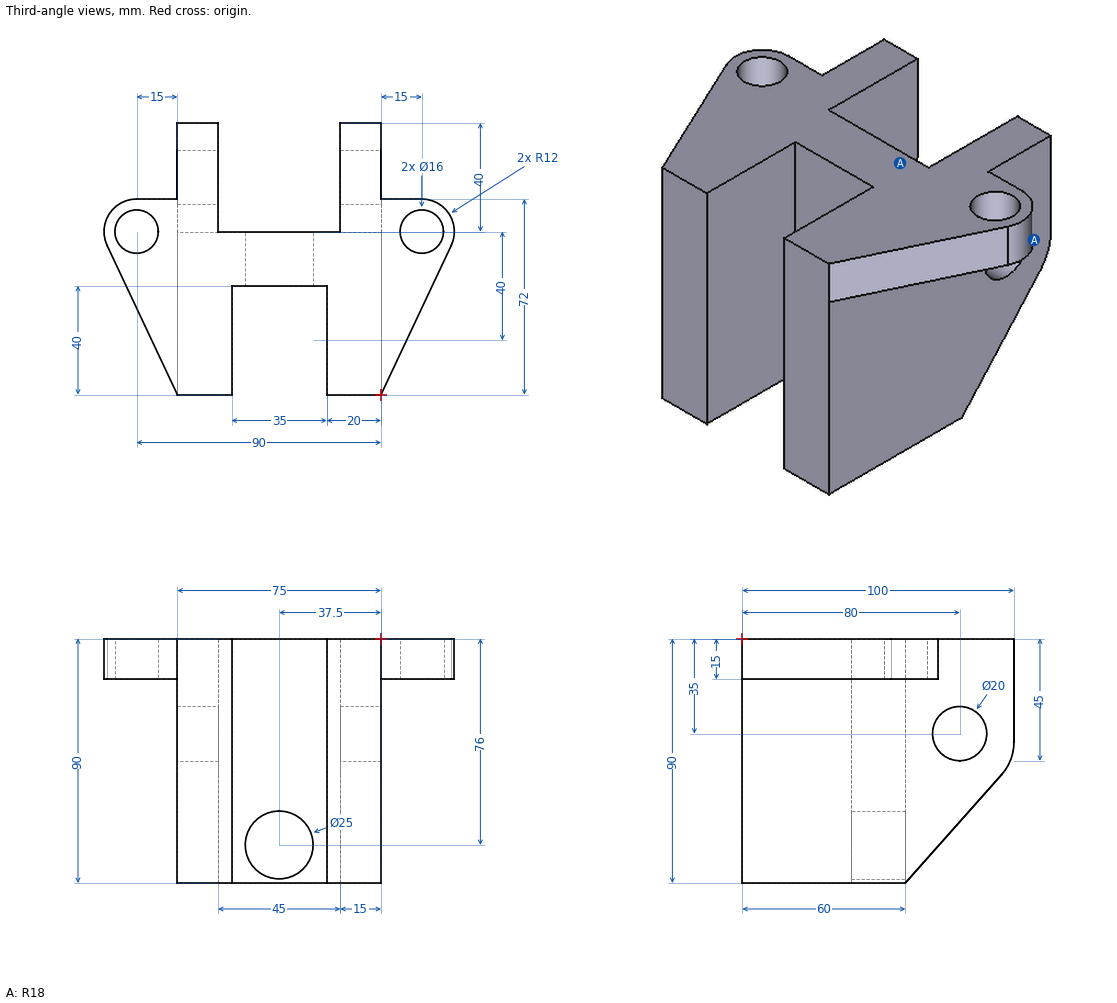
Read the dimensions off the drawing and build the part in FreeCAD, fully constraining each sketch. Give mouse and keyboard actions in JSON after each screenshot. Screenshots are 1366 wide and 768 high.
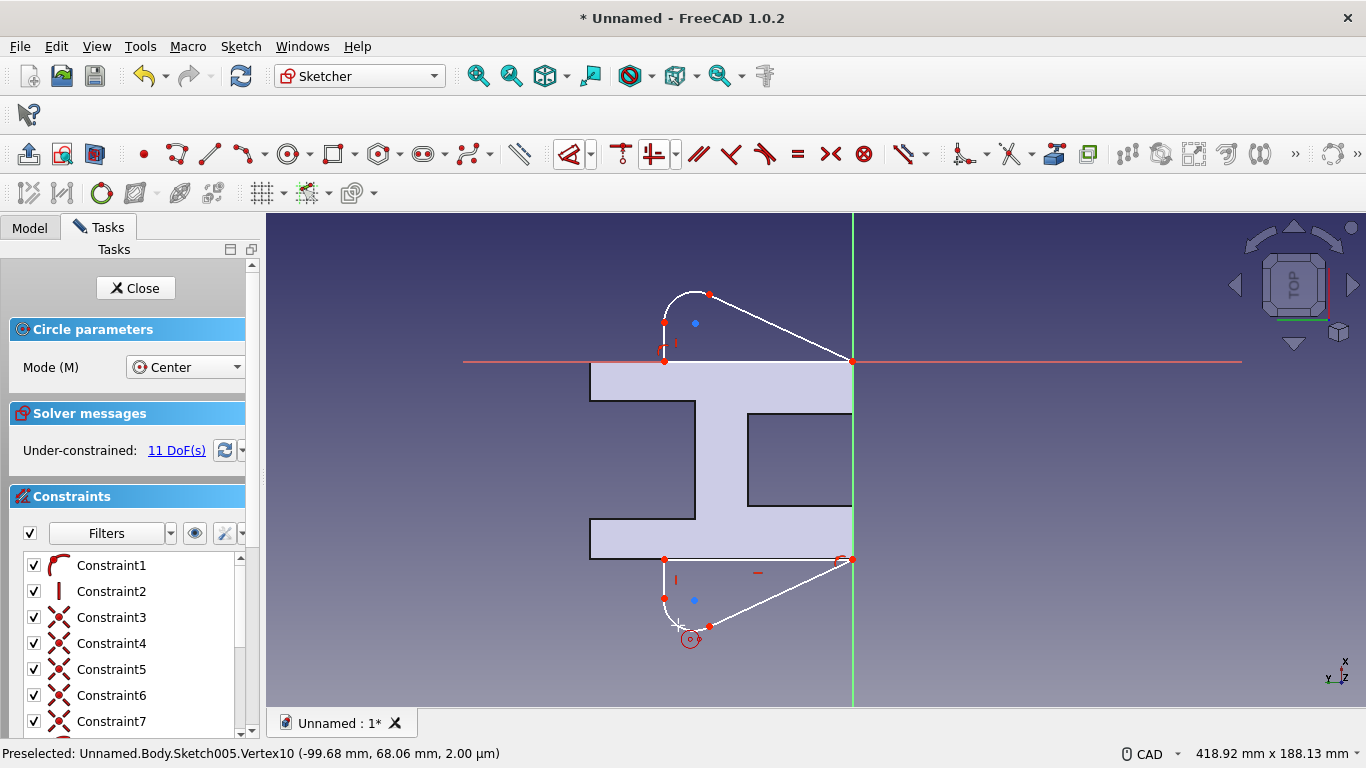
{"action": "left_click", "coordinate": [695, 322]}
{"action": "left_click", "coordinate": [710, 337]}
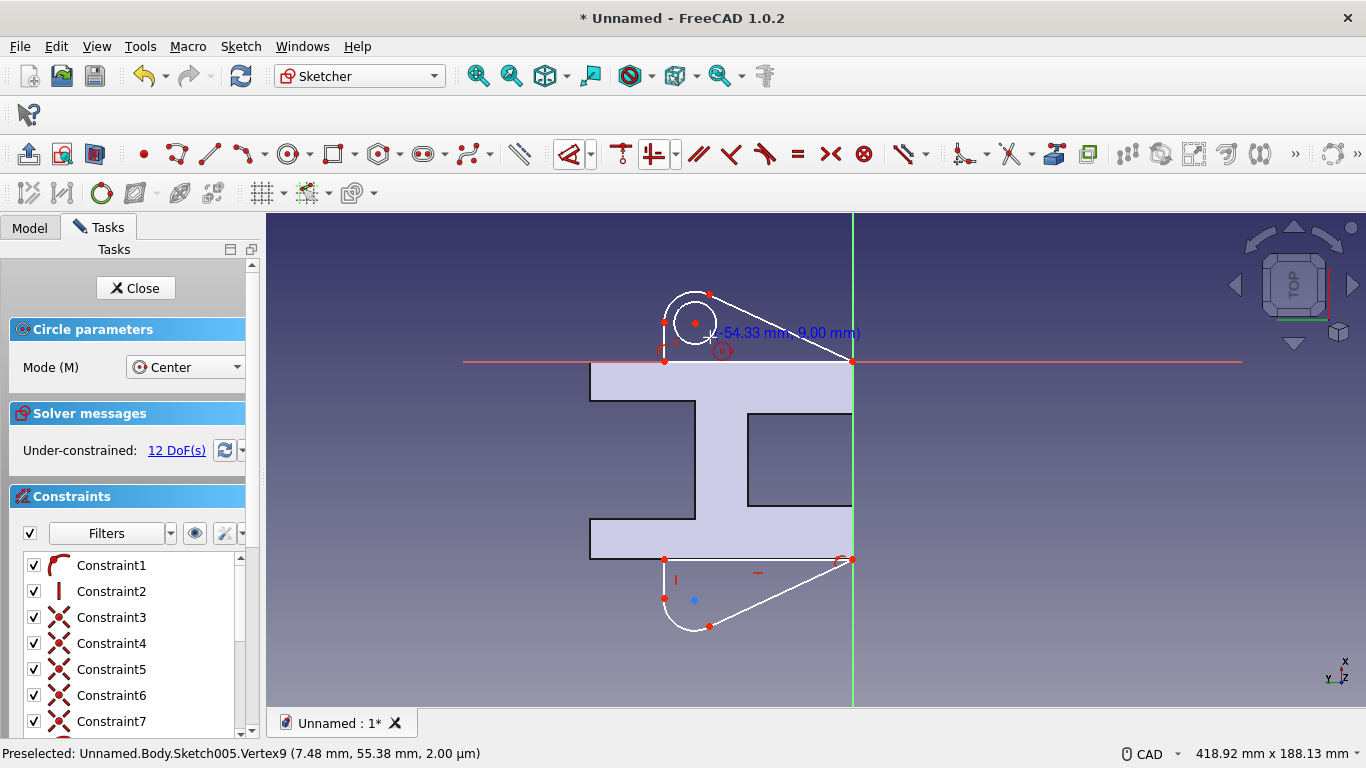
{"action": "left_click", "coordinate": [695, 598]}
{"action": "left_click", "coordinate": [710, 583]}
{"action": "key", "text": "Escape"}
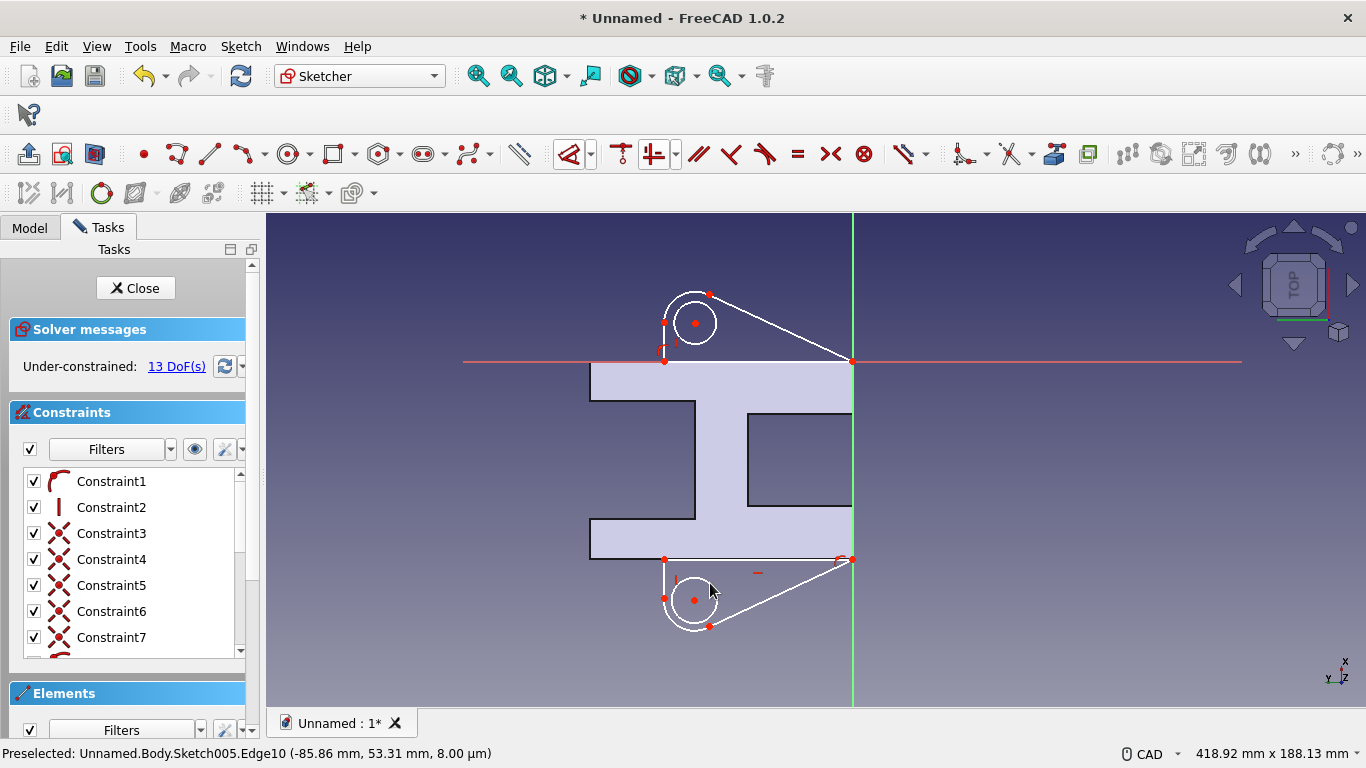
{"action": "left_click", "coordinate": [664, 335]}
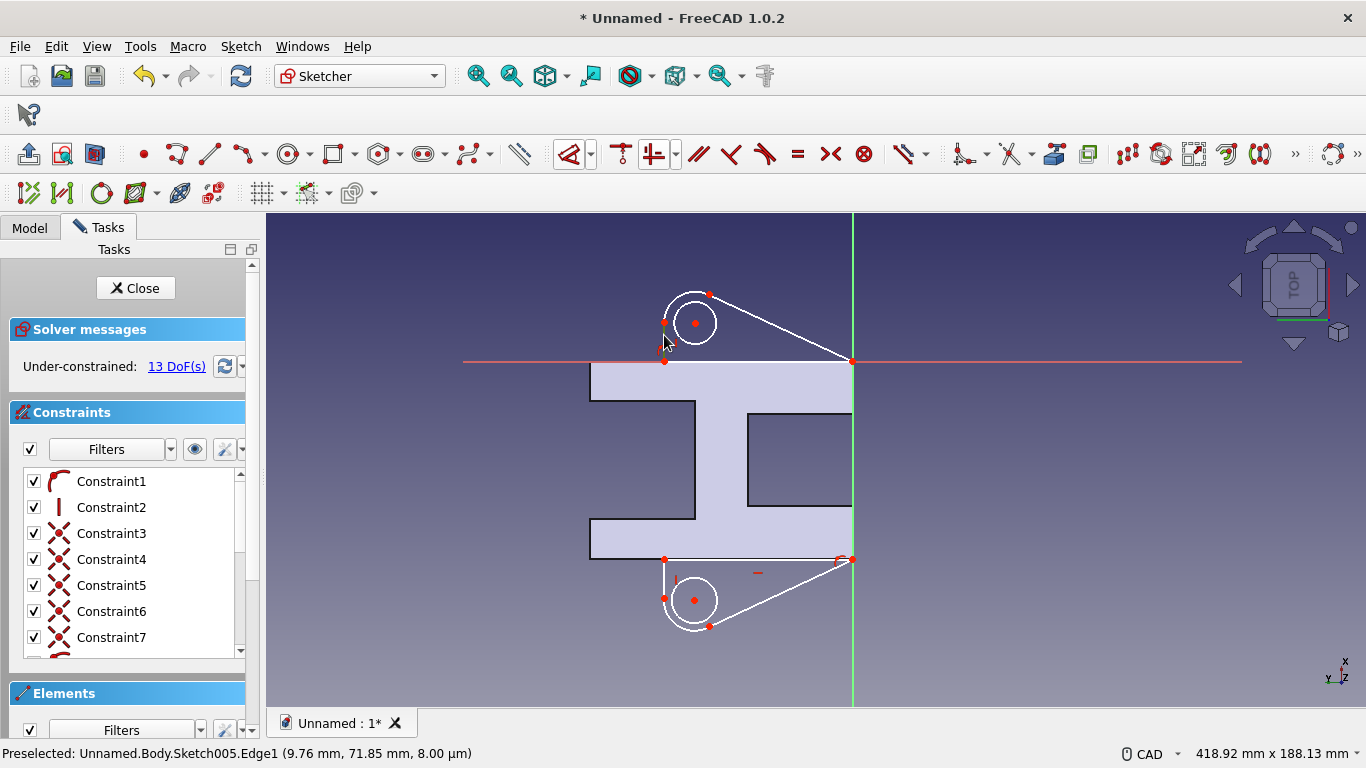
{"action": "scroll", "coordinate": [691, 292], "scroll_direction": "up", "scroll_amount": 2}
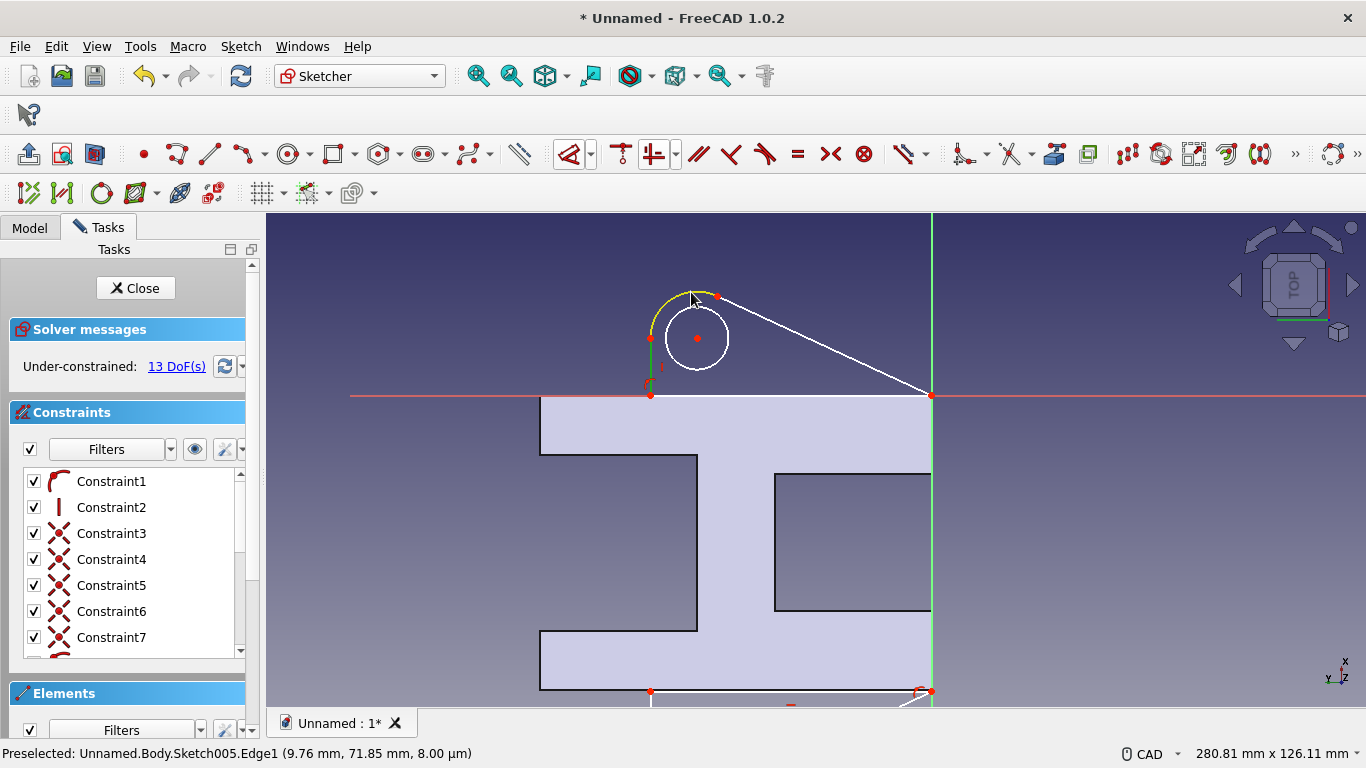
{"action": "left_click", "coordinate": [690, 292]}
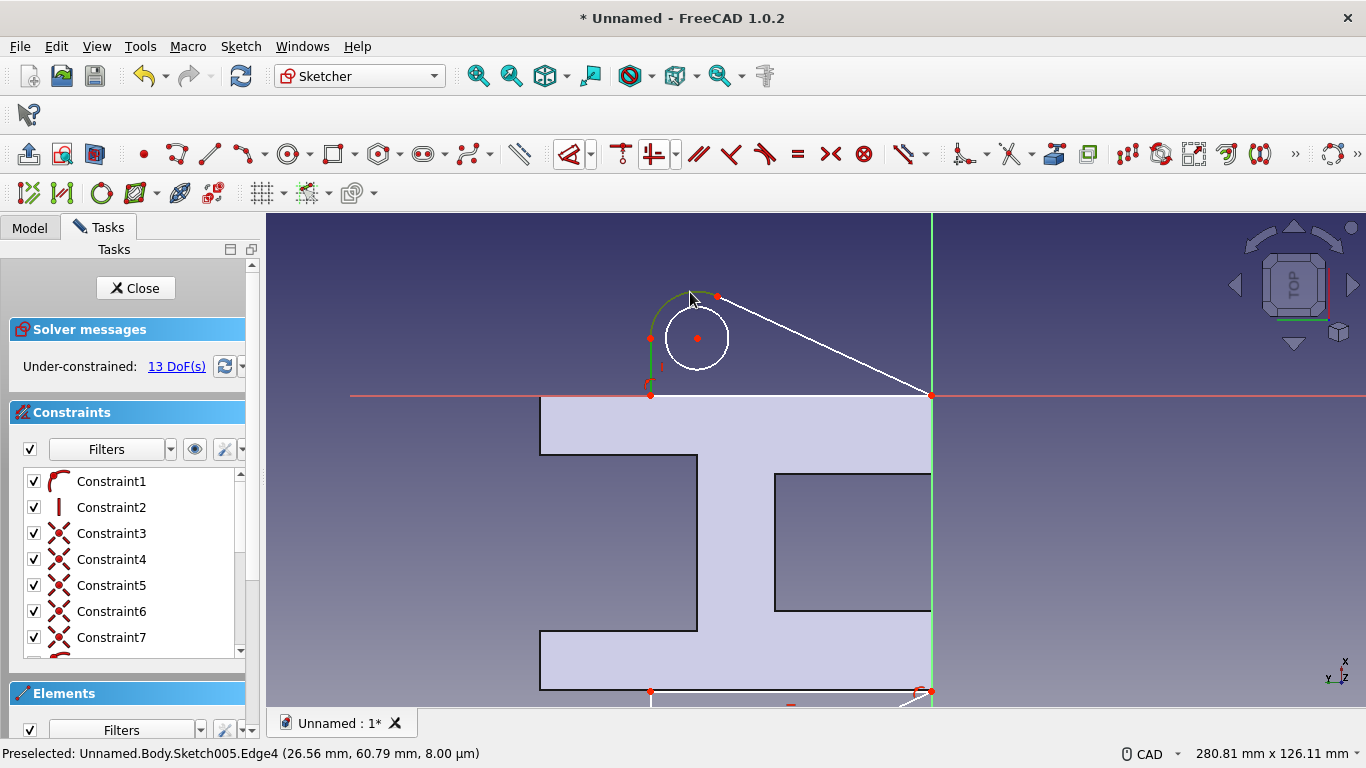
{"action": "left_click", "coordinate": [765, 154]}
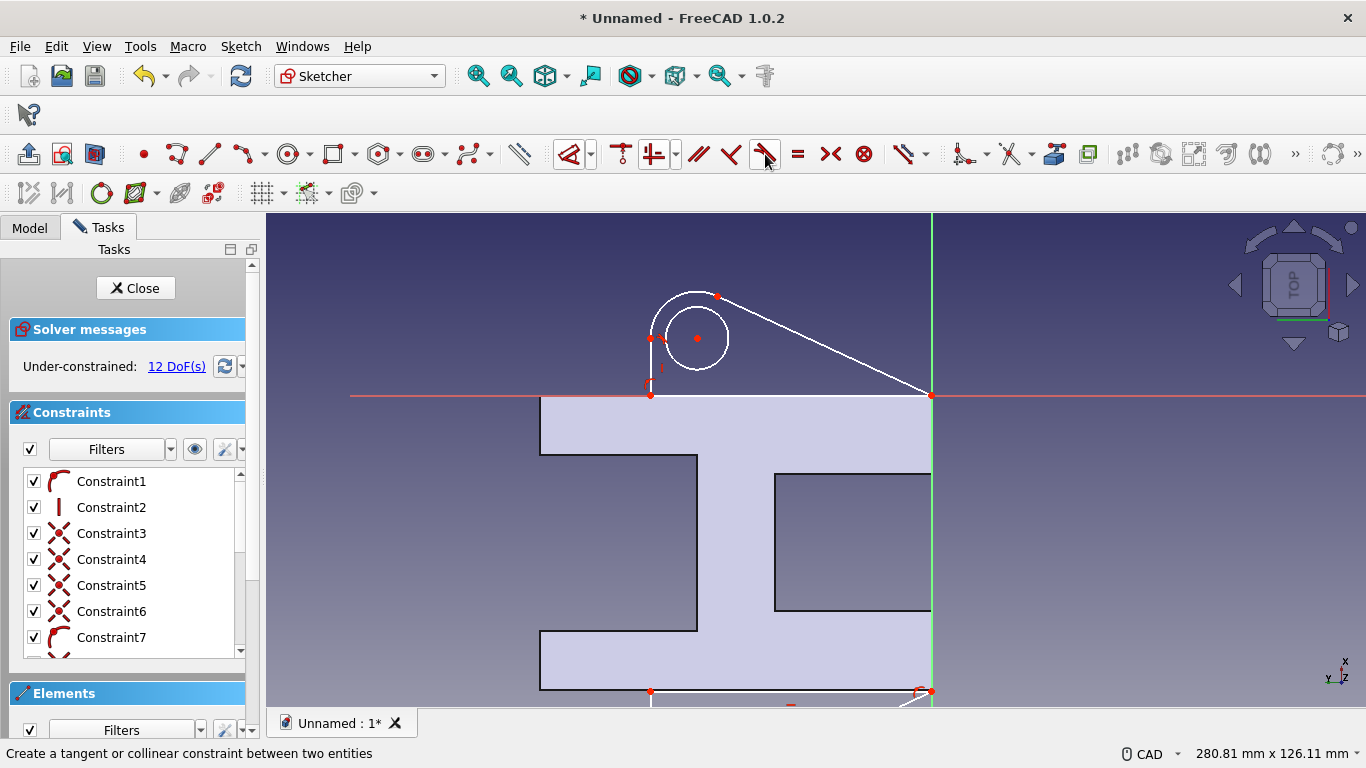
{"action": "left_click", "coordinate": [868, 366]}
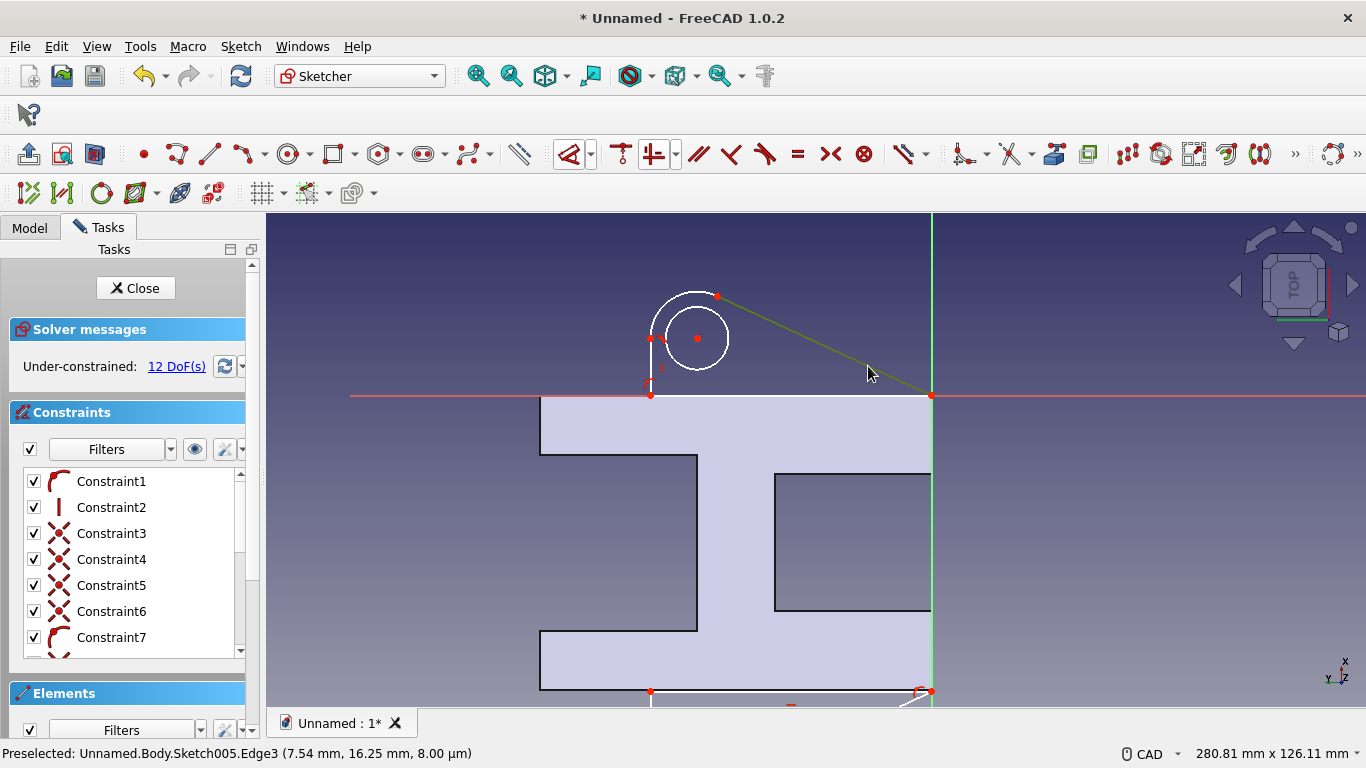
{"action": "left_click", "coordinate": [690, 292]}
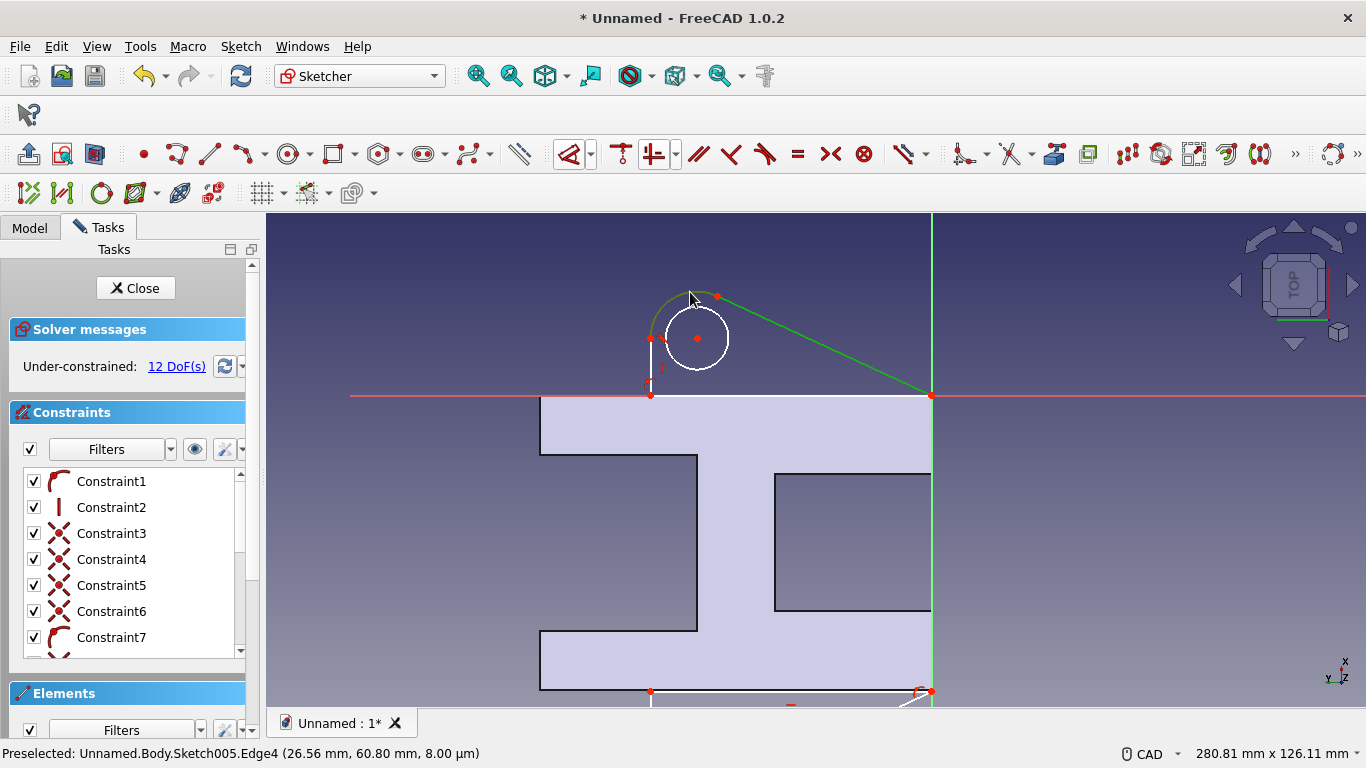
{"action": "left_click", "coordinate": [765, 154]}